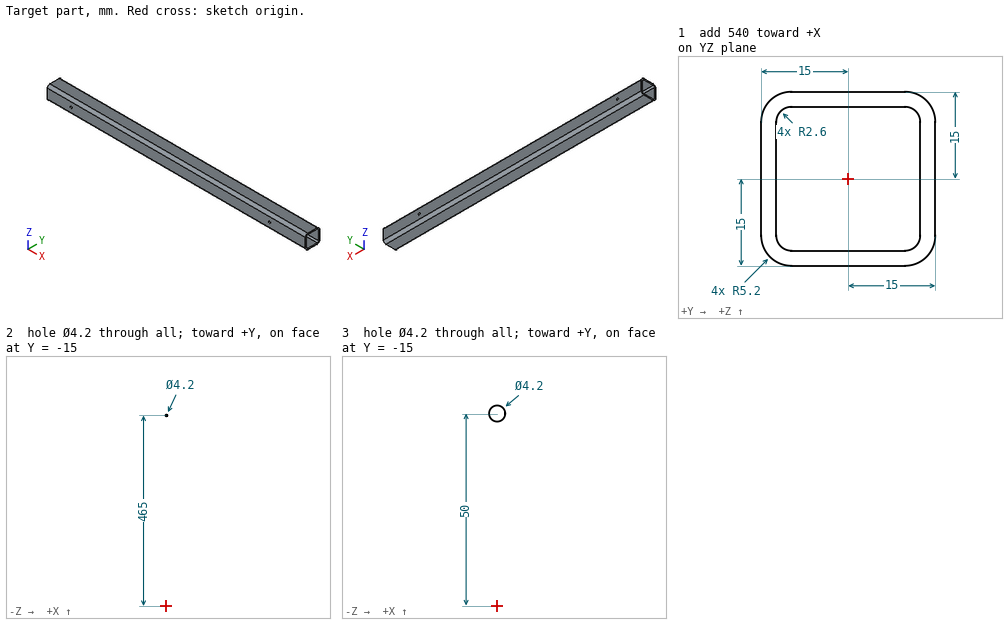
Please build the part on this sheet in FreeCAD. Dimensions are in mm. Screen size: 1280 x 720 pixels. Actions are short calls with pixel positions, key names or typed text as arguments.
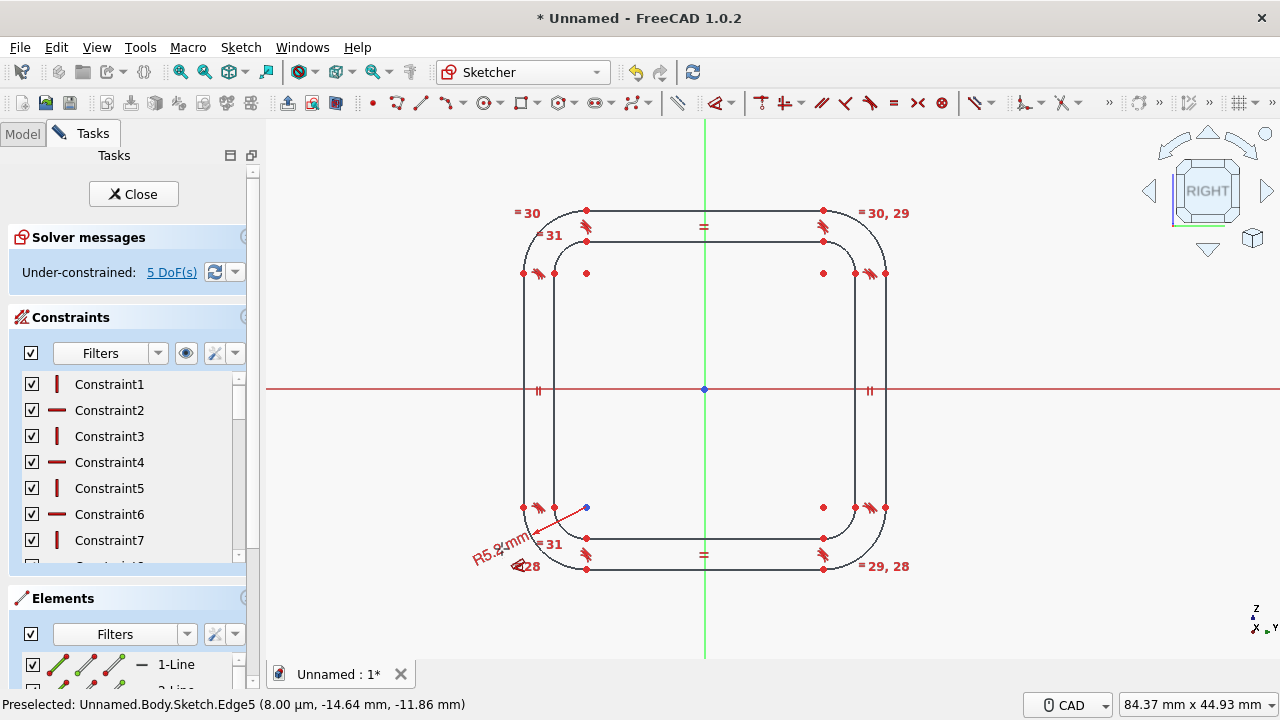
scroll(572, 245, up, 2)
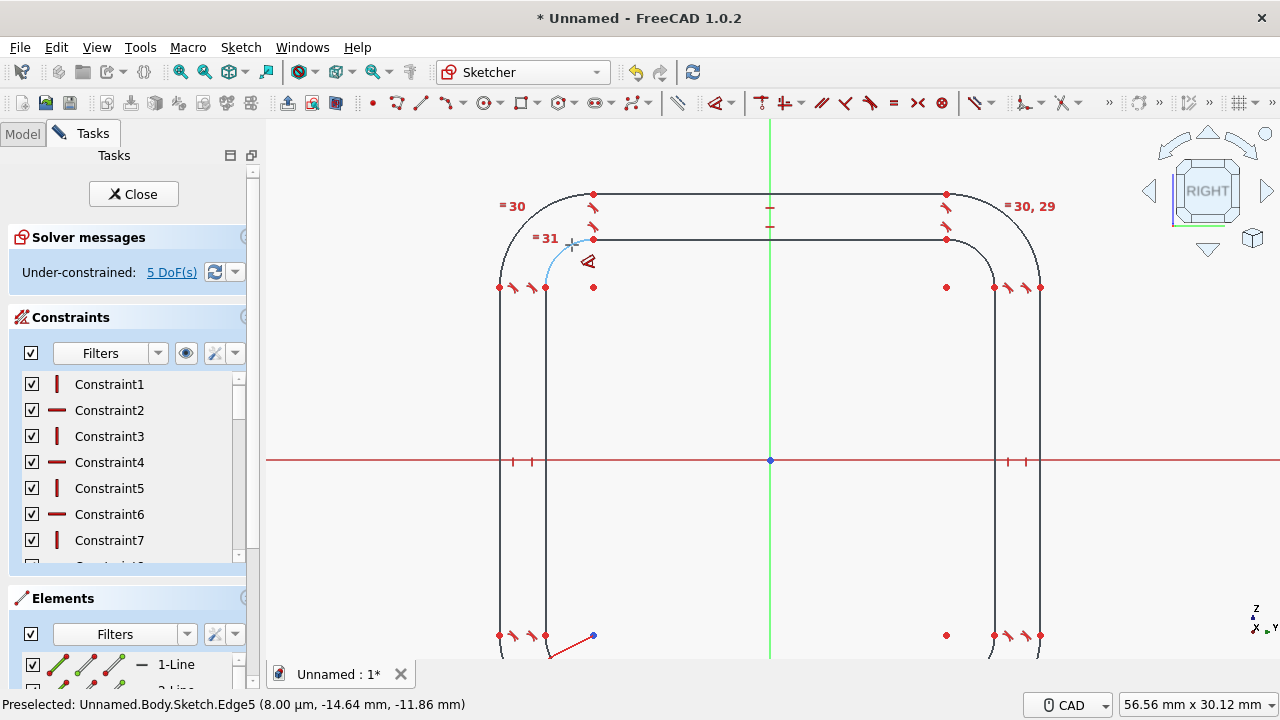
click(572, 245)
click(558, 216)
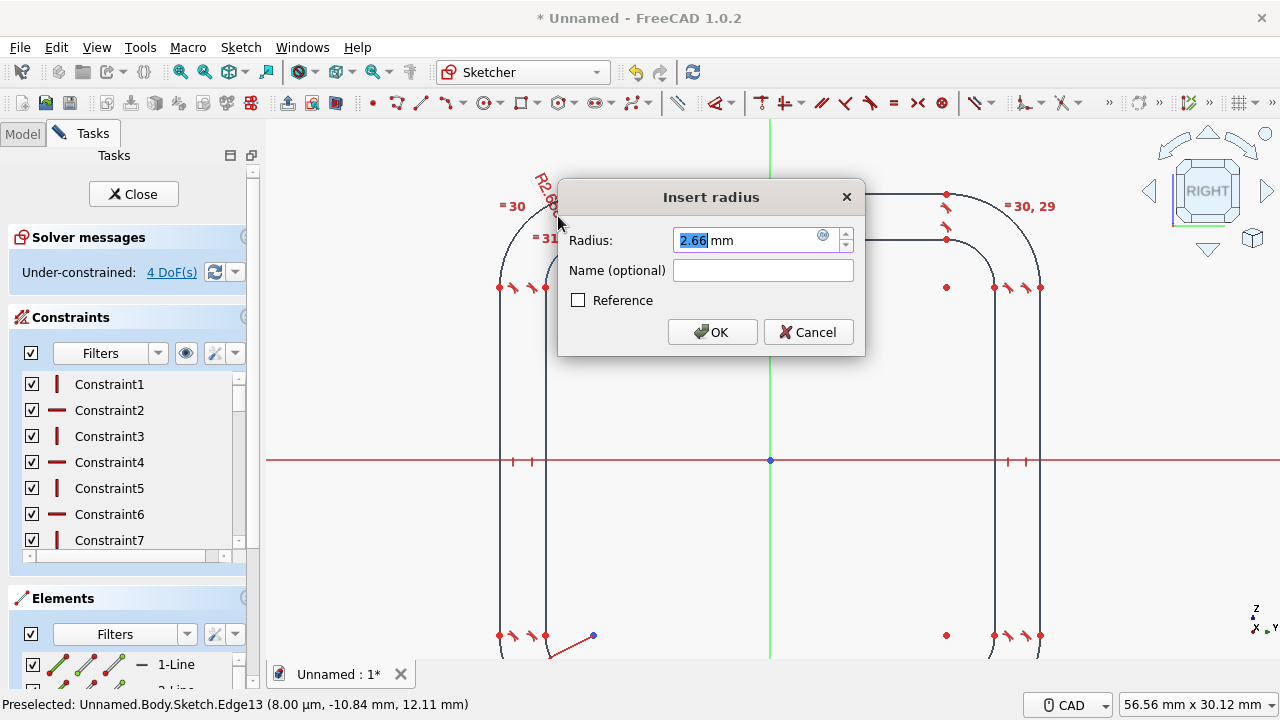
text(2.6)
key(Return)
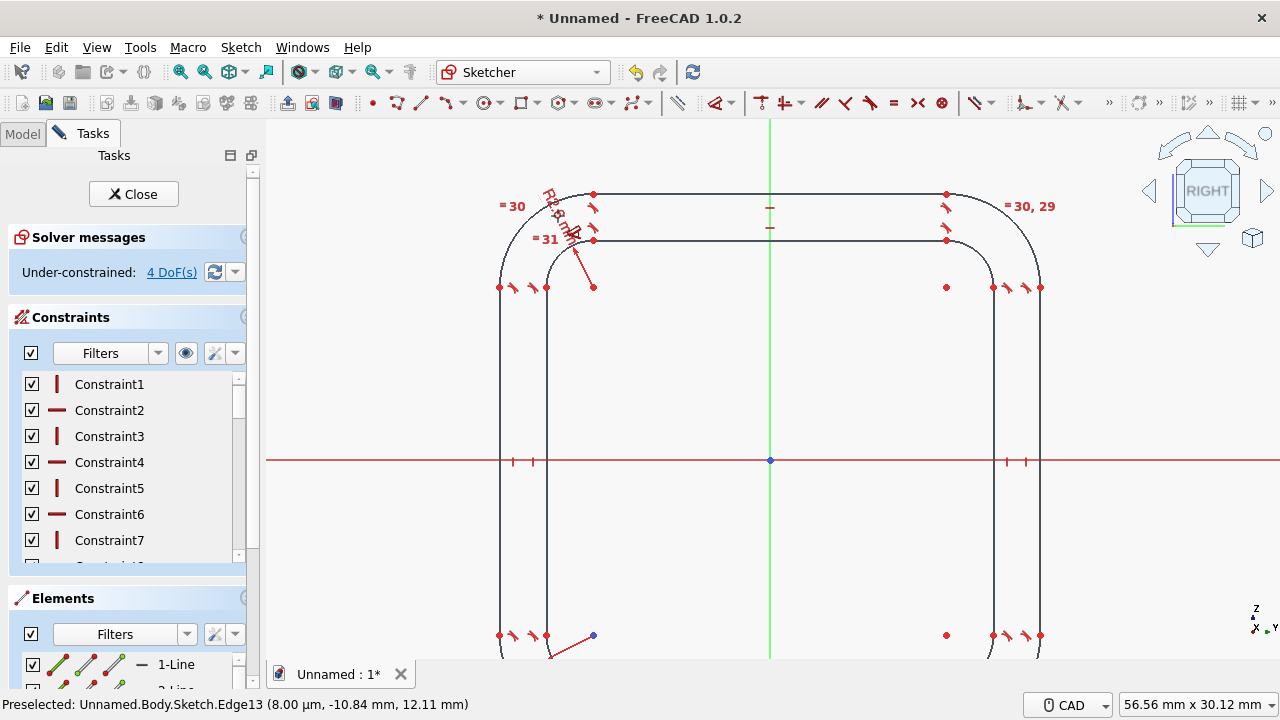
click(500, 287)
click(540, 253)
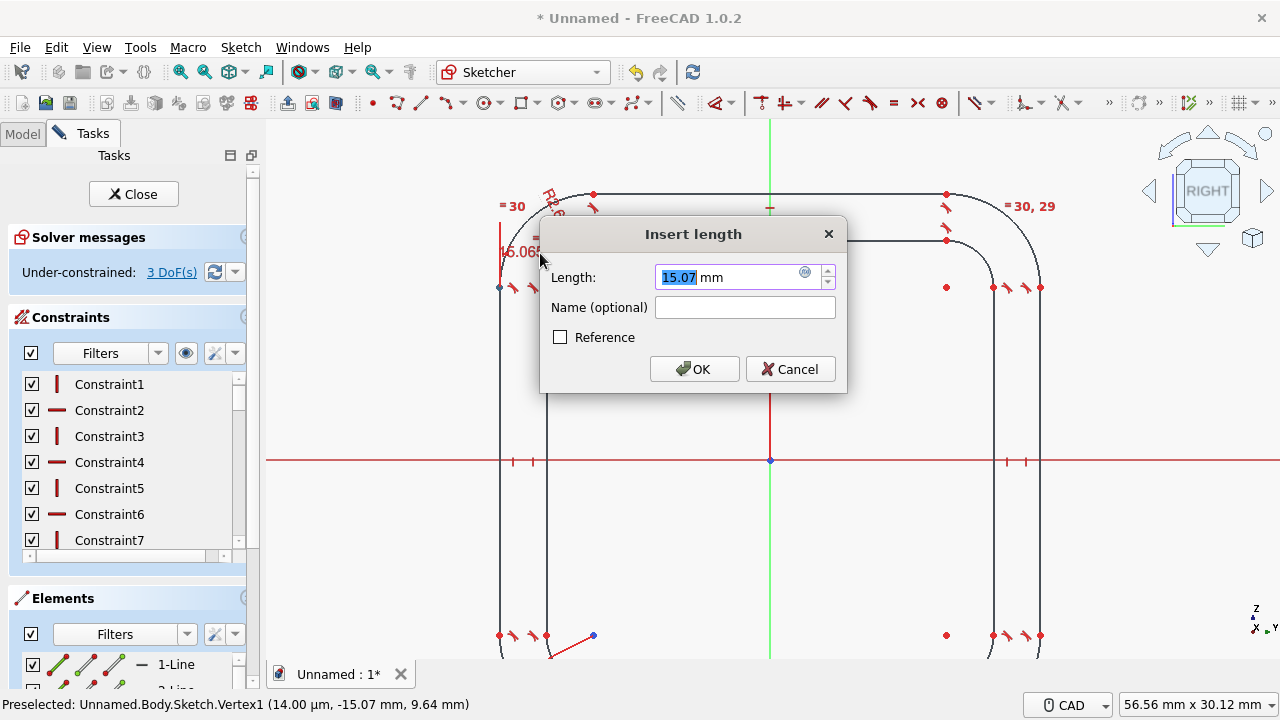
text(15)
key(Return)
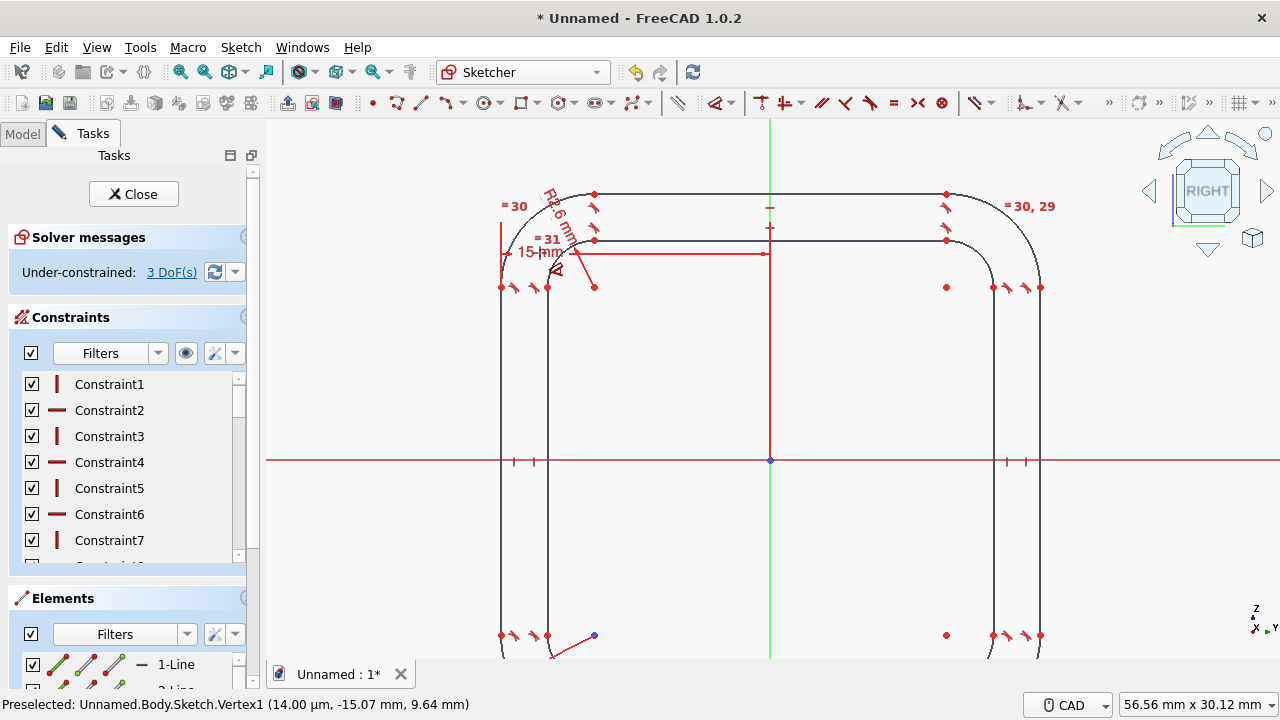
scroll(571, 244, down, 2)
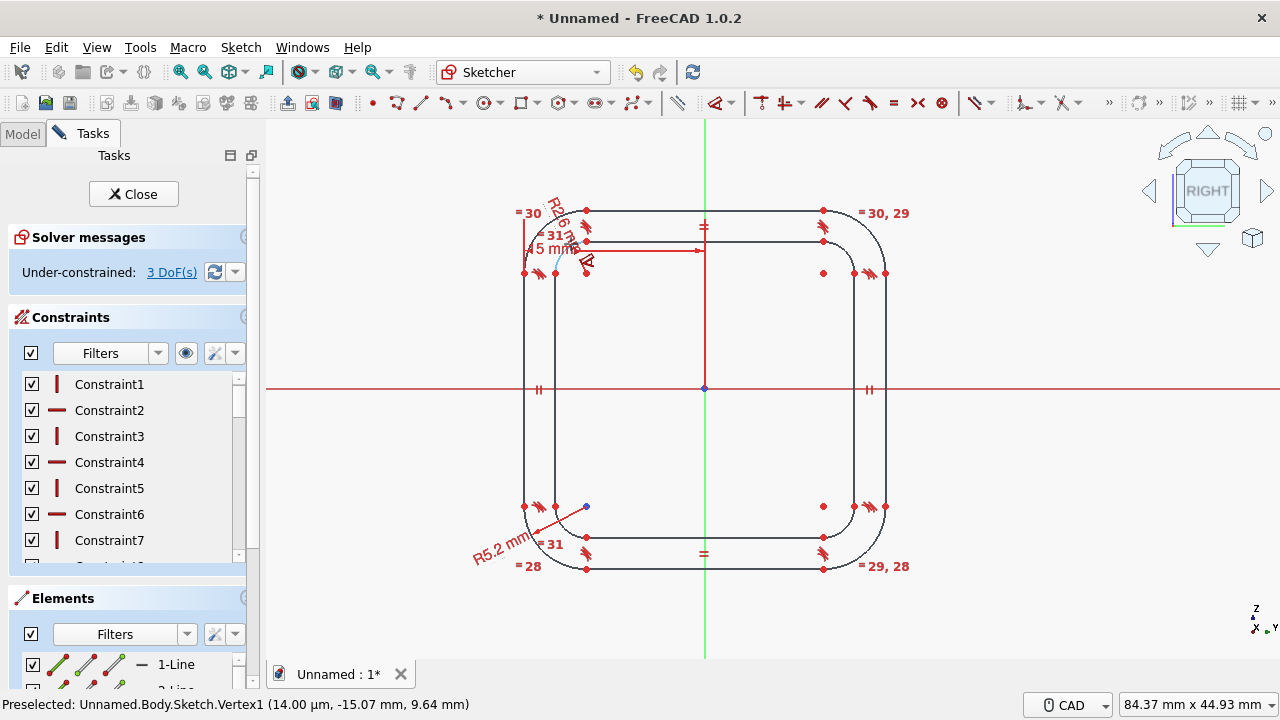
click(587, 569)
click(739, 479)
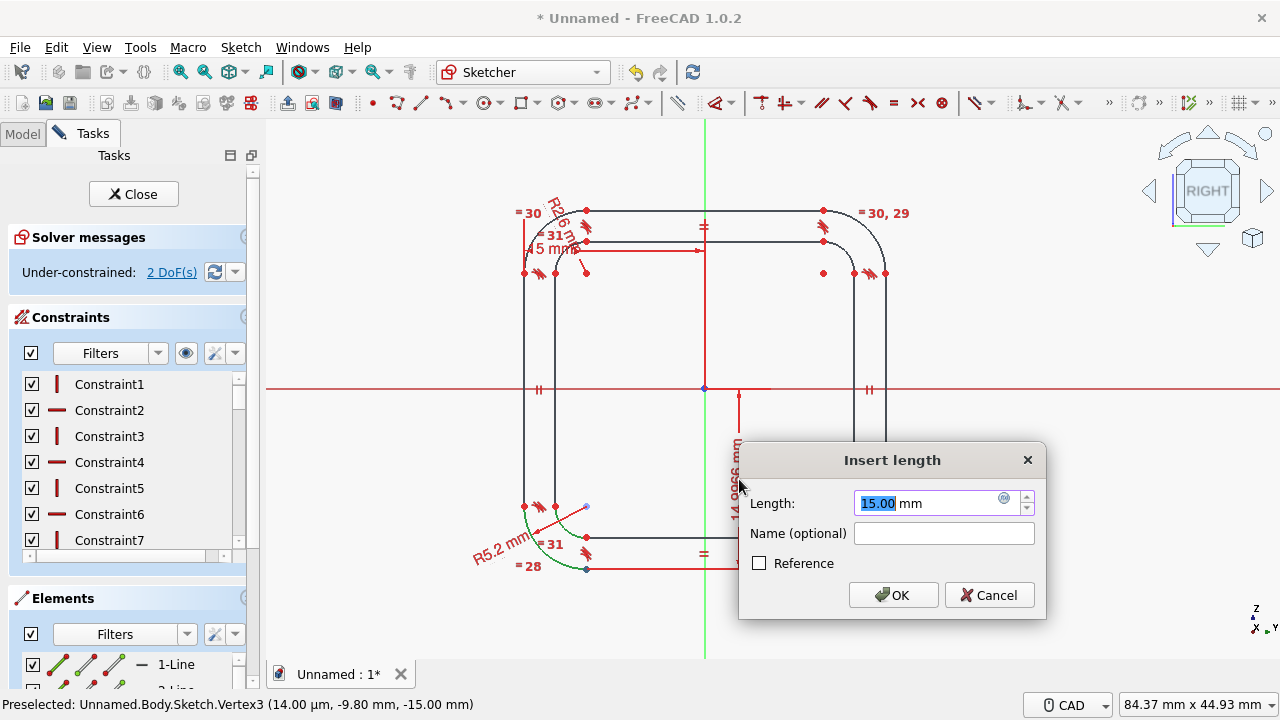
text(15)
key(Return)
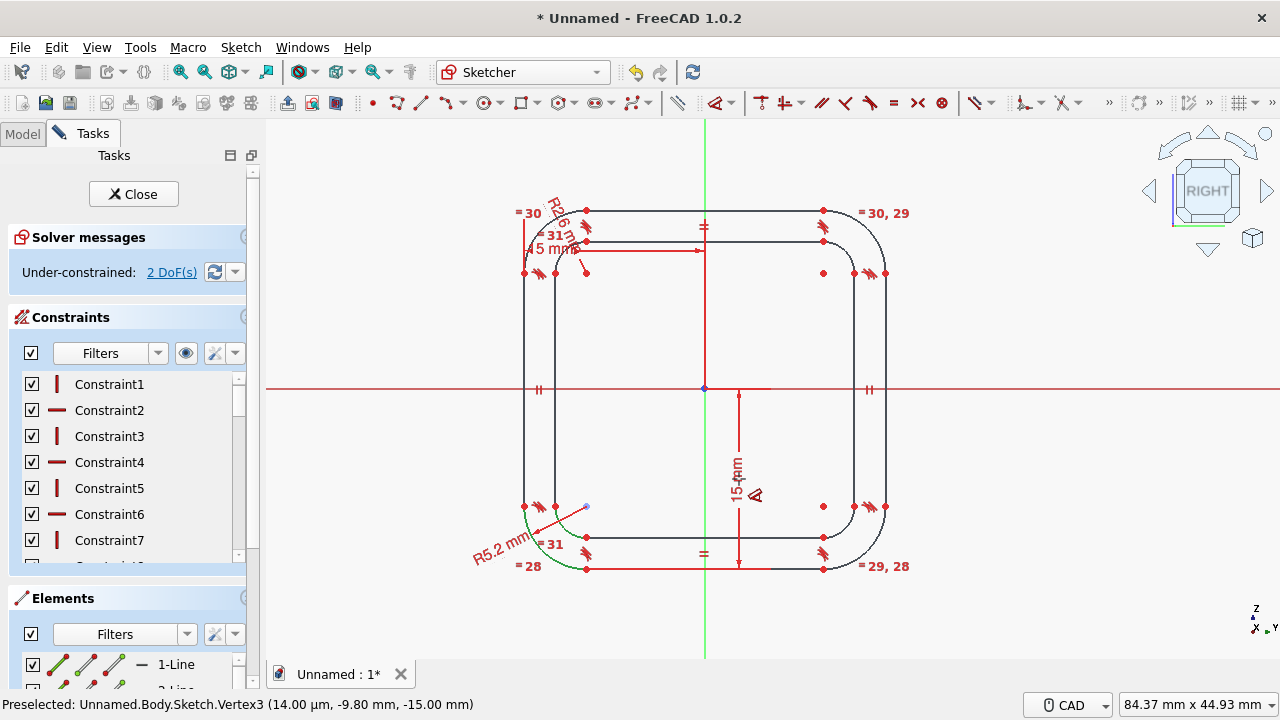
click(886, 507)
click(858, 541)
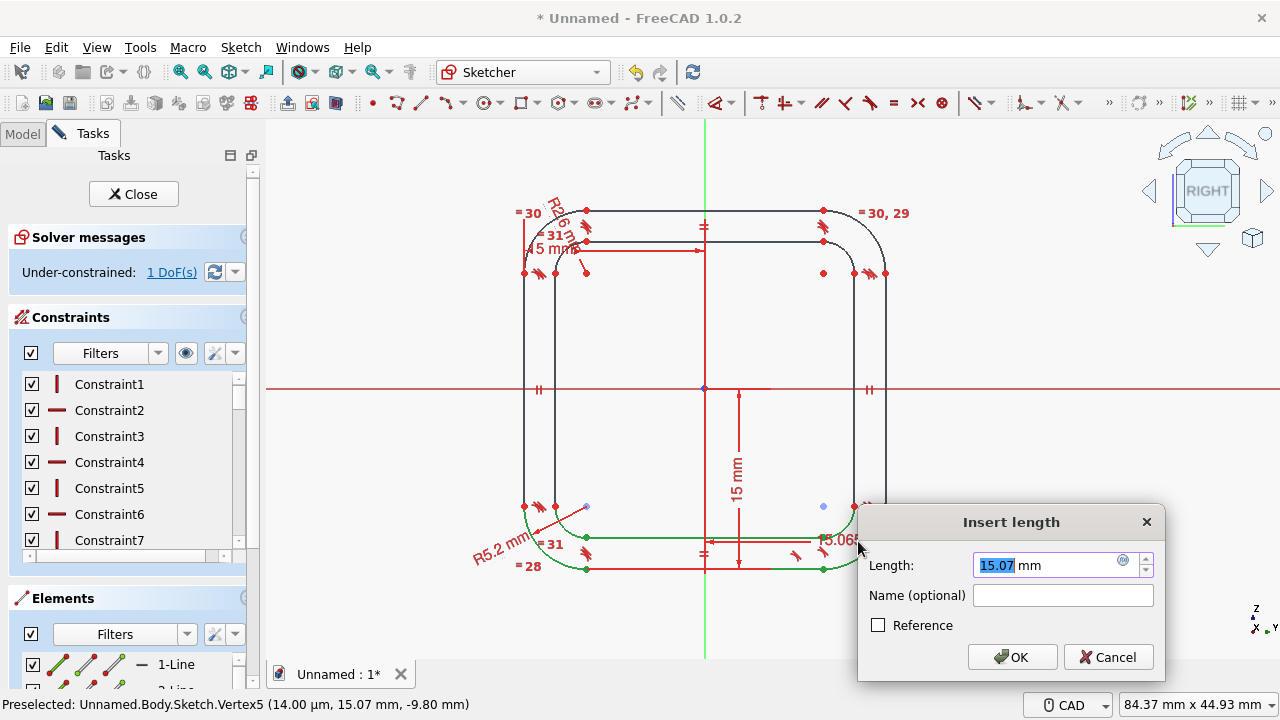
text(15)
key(Return)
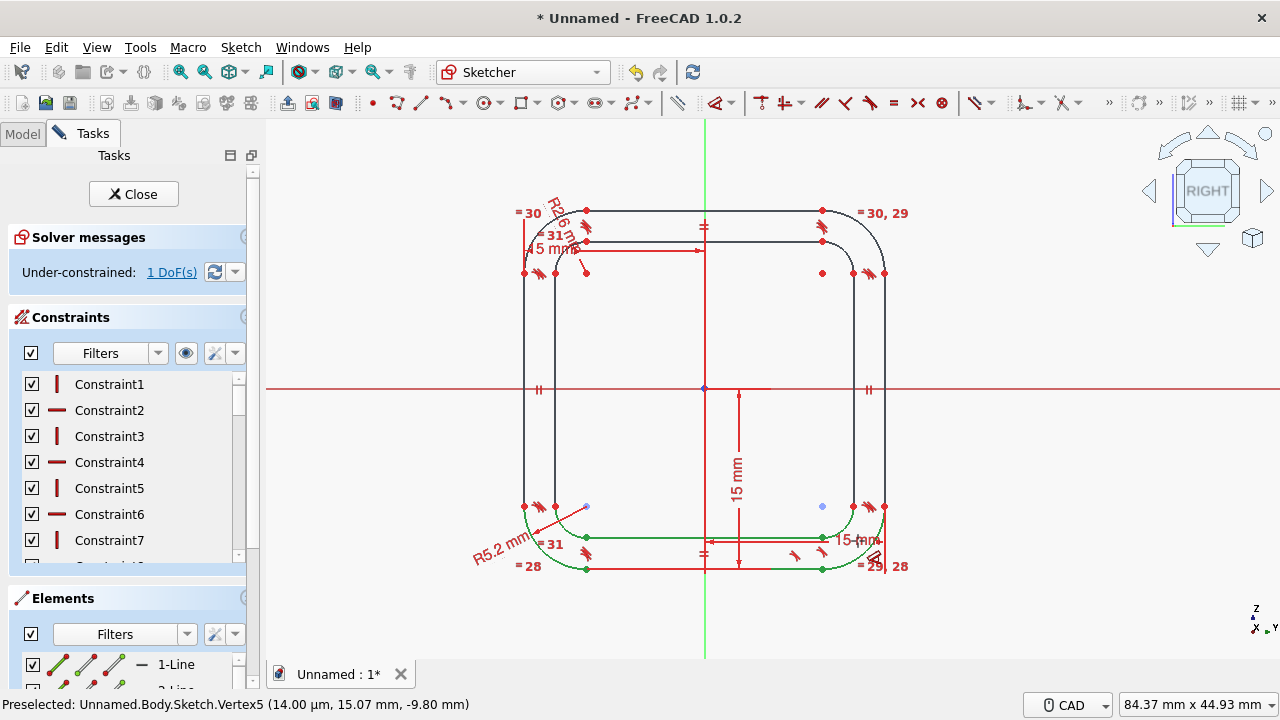
click(822, 211)
click(856, 237)